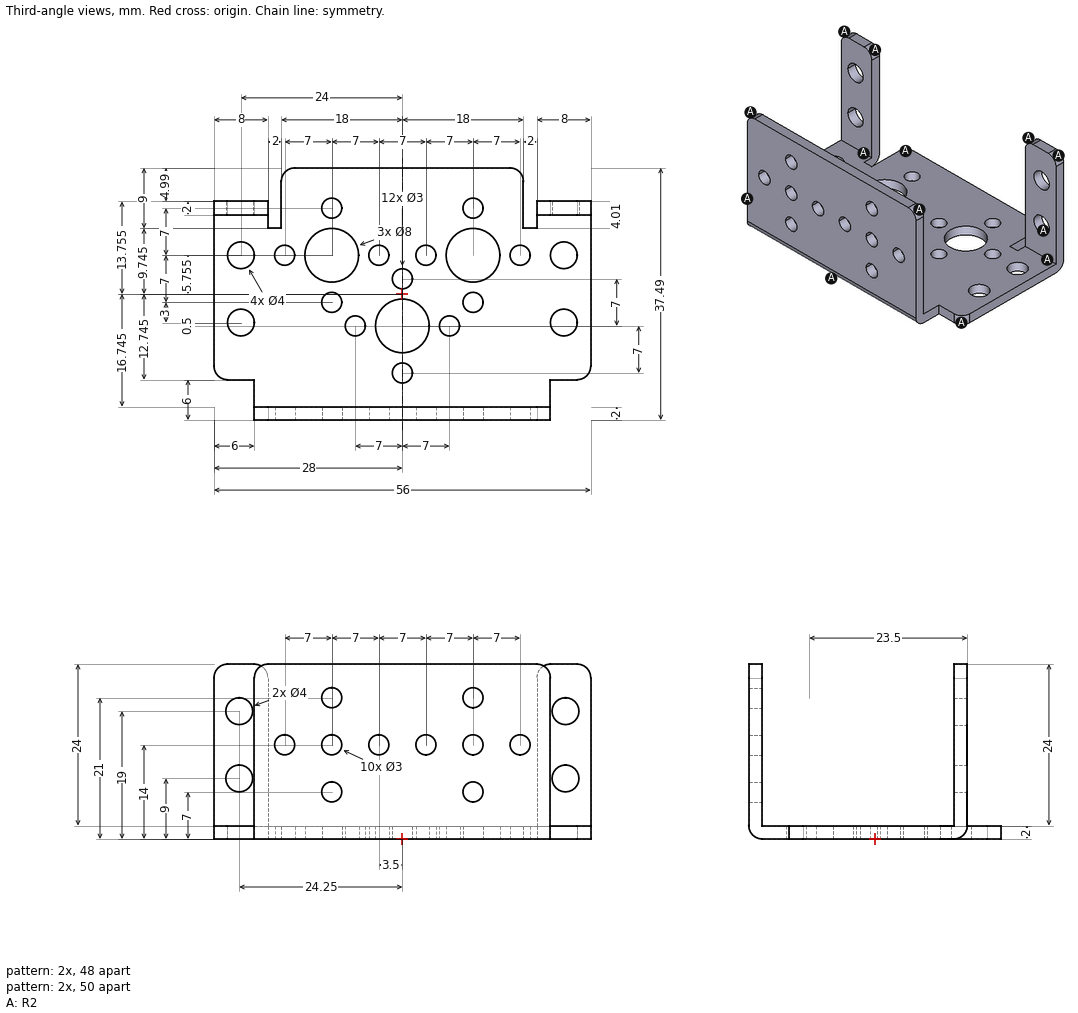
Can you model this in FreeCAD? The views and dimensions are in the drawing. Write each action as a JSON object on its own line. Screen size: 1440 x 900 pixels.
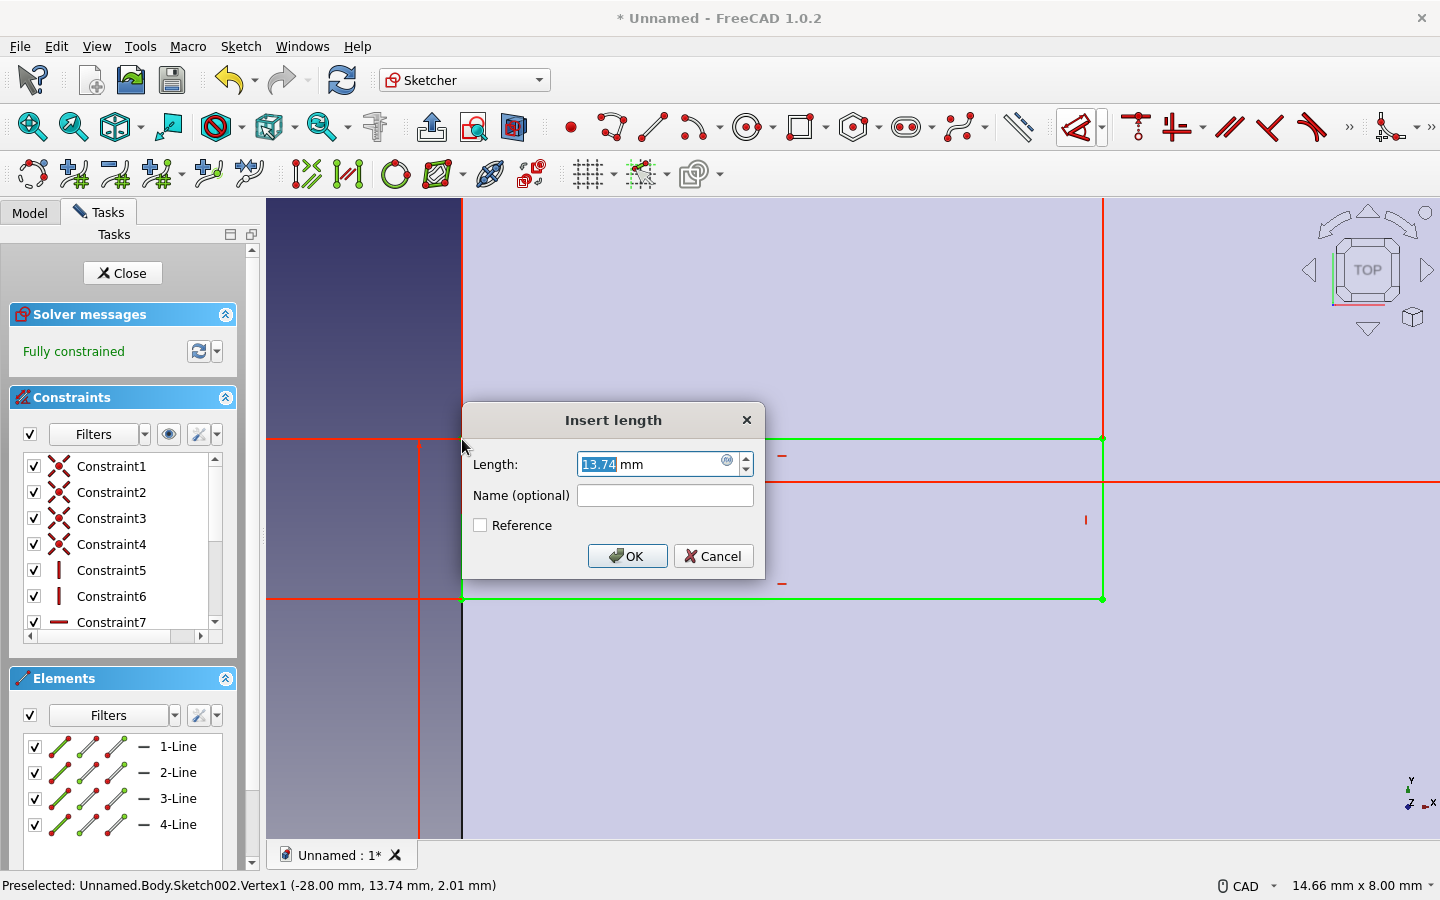
{"action": "type", "text": "13.755"}
{"action": "key", "text": "Return"}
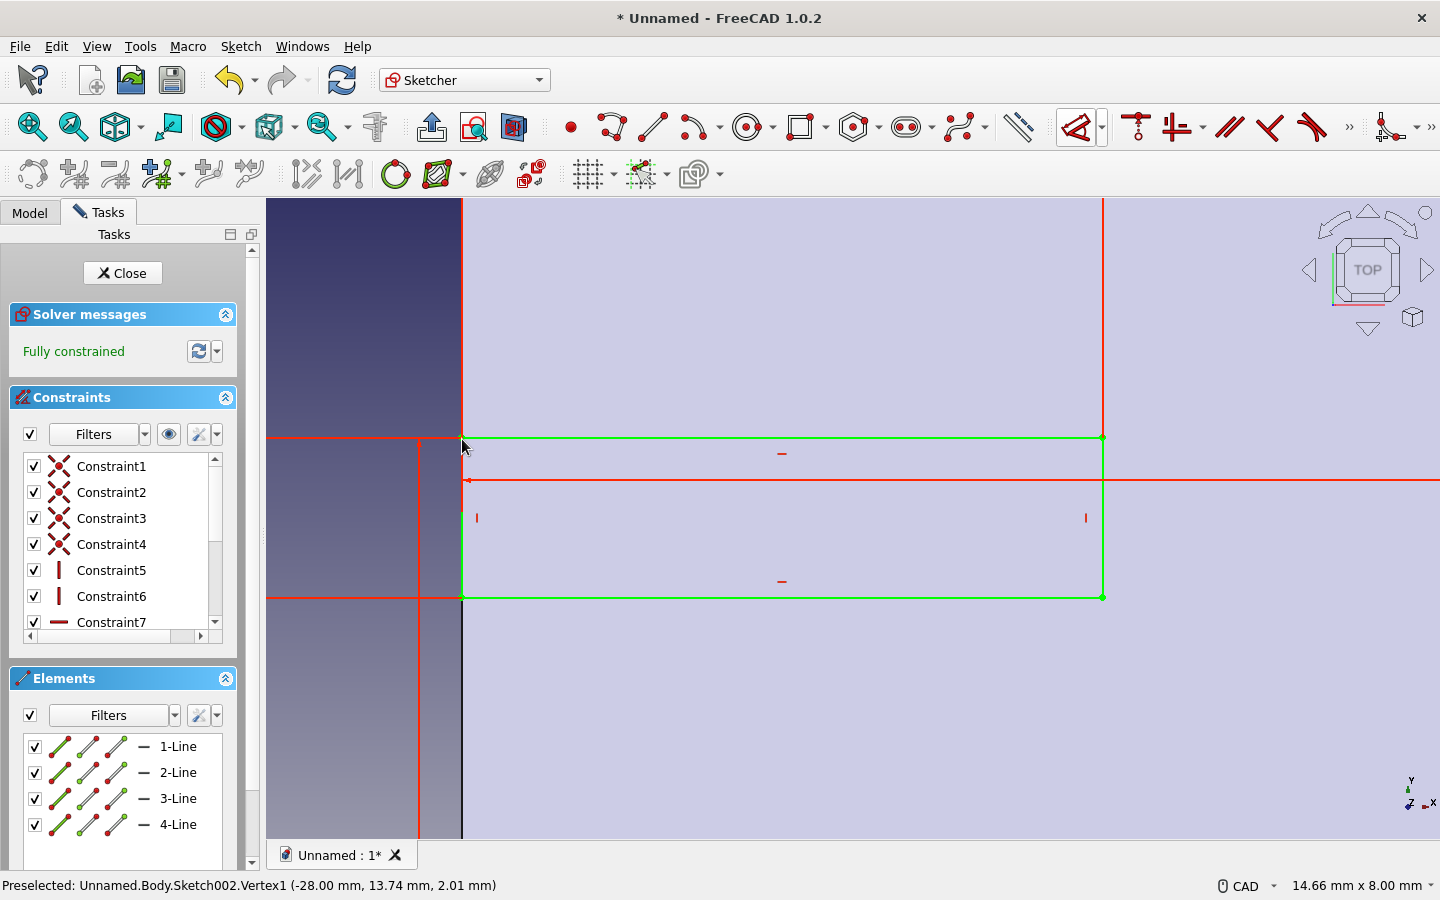
{"action": "left_click", "coordinate": [123, 273]}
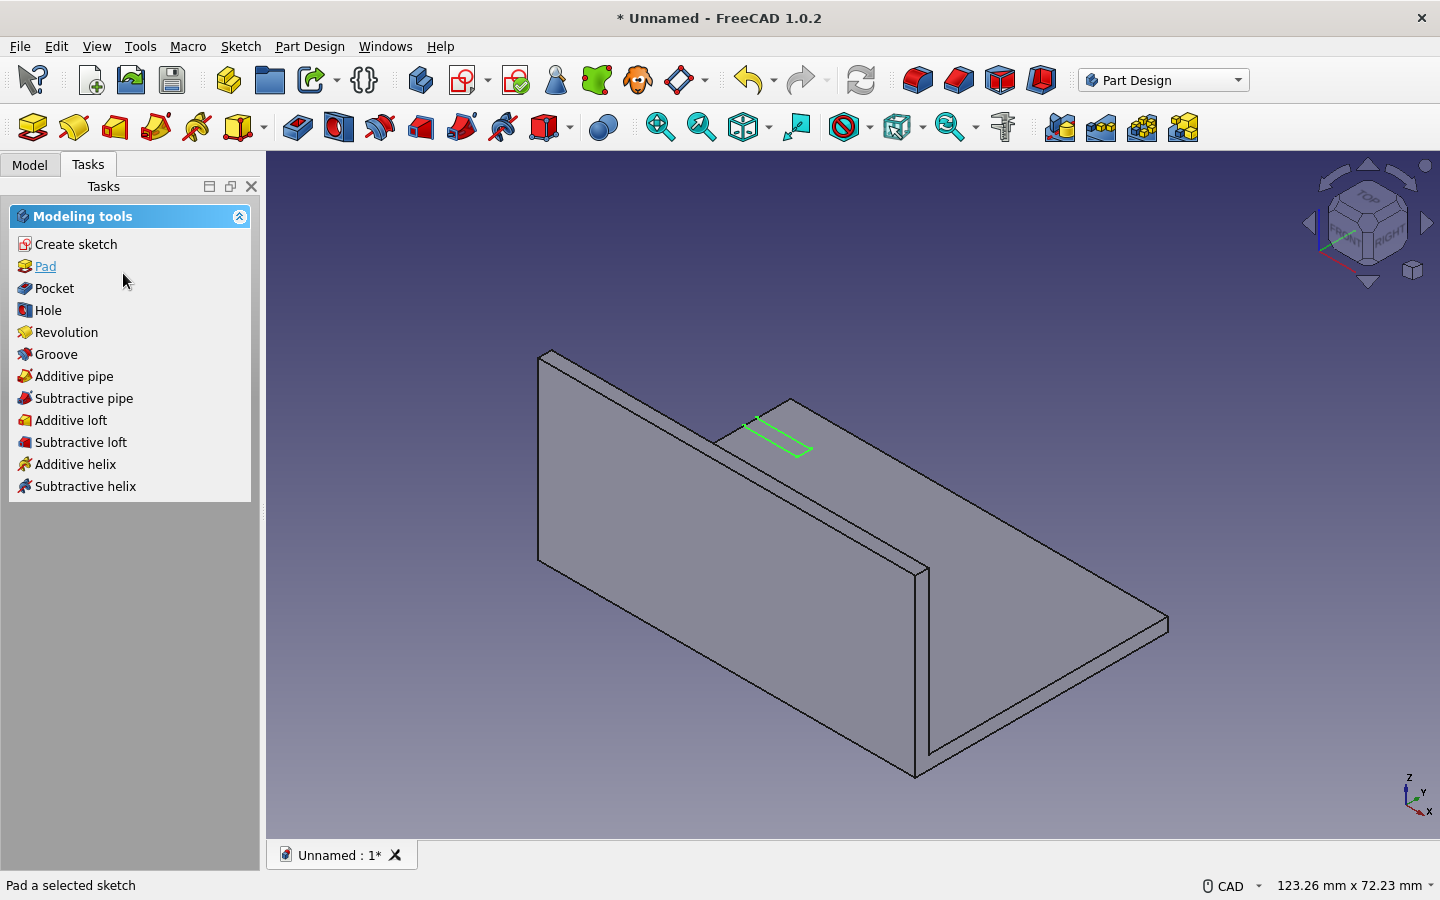
{"action": "left_click", "coordinate": [33, 128]}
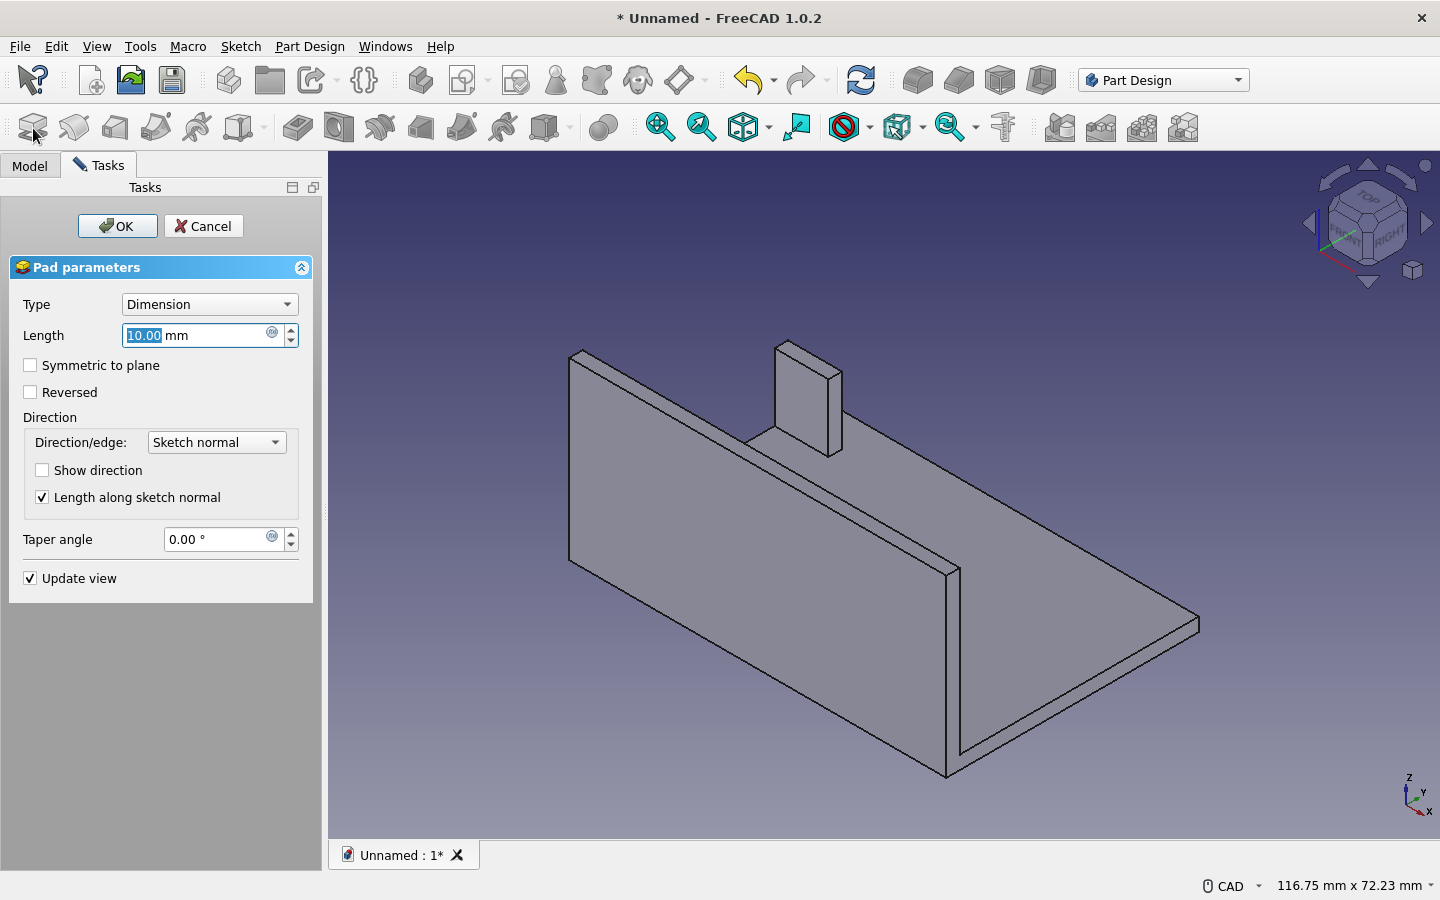
{"action": "type", "text": "24"}
{"action": "key", "text": "Tab"}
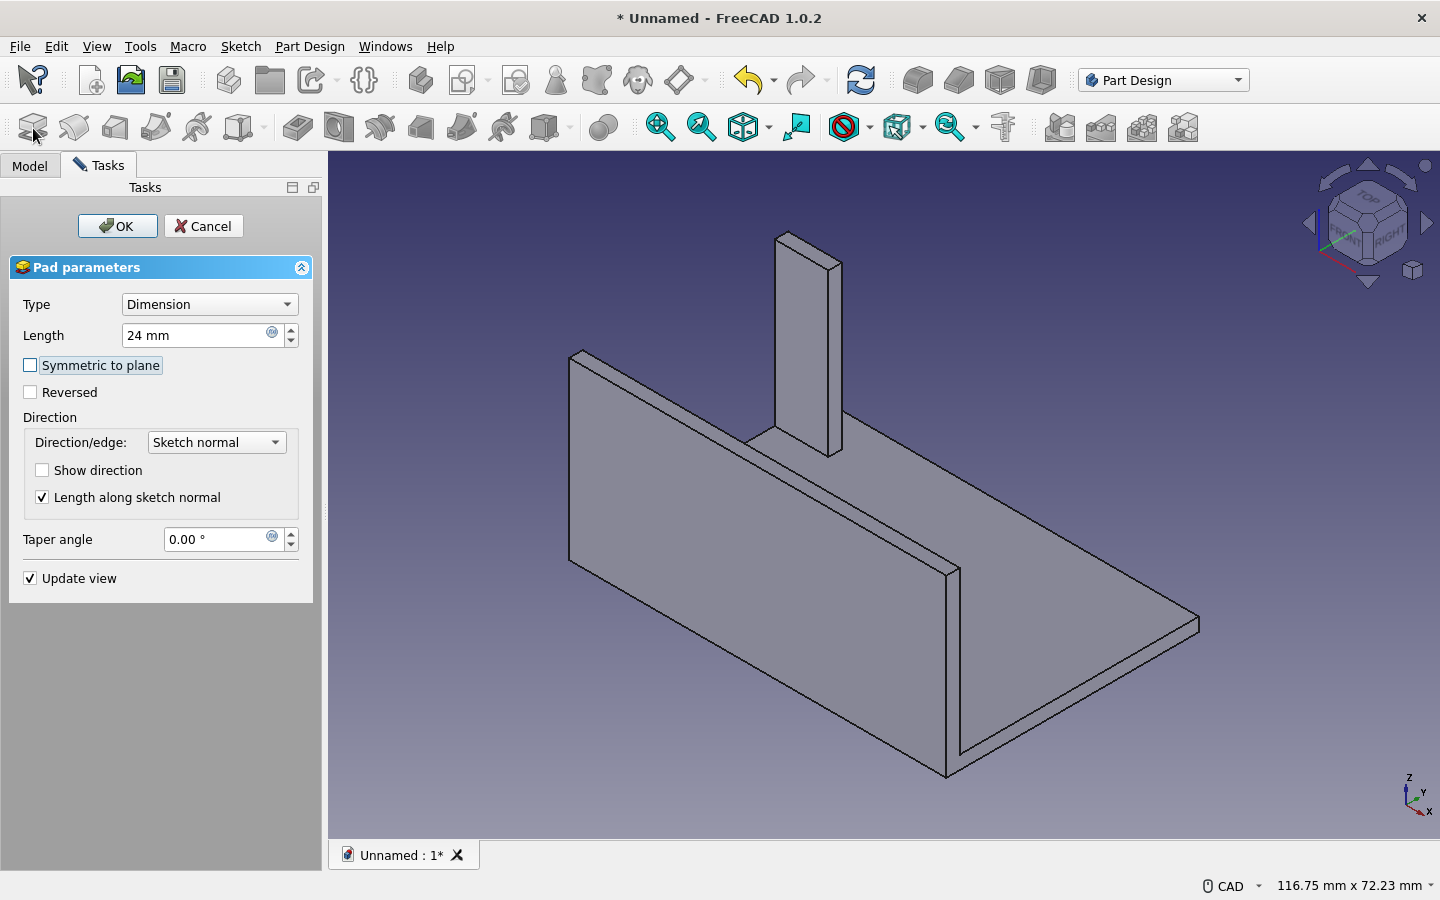
{"action": "left_click", "coordinate": [118, 226]}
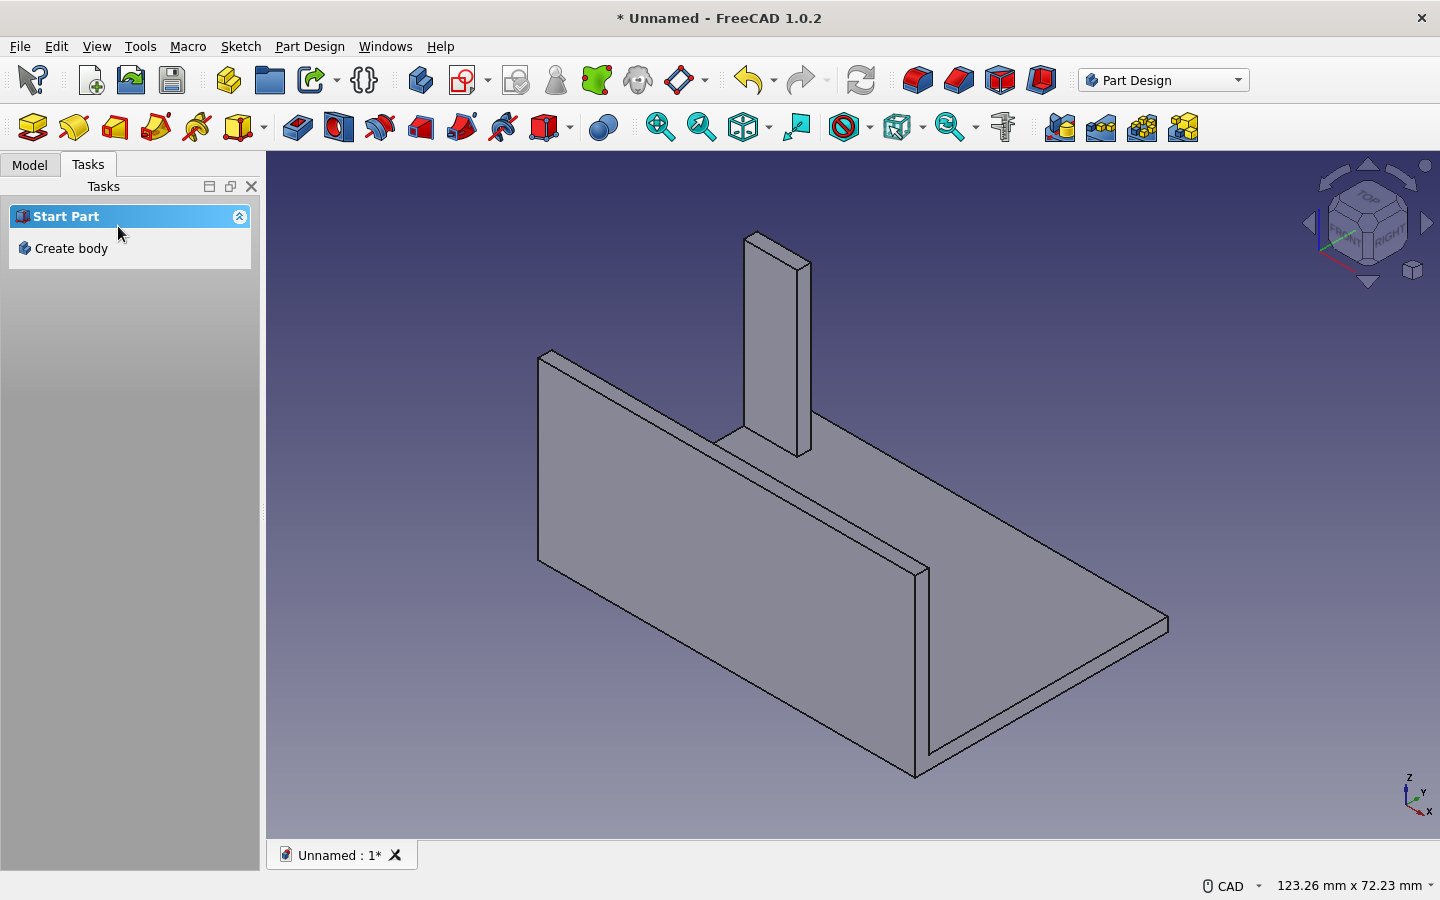
{"action": "left_click", "coordinate": [30, 164]}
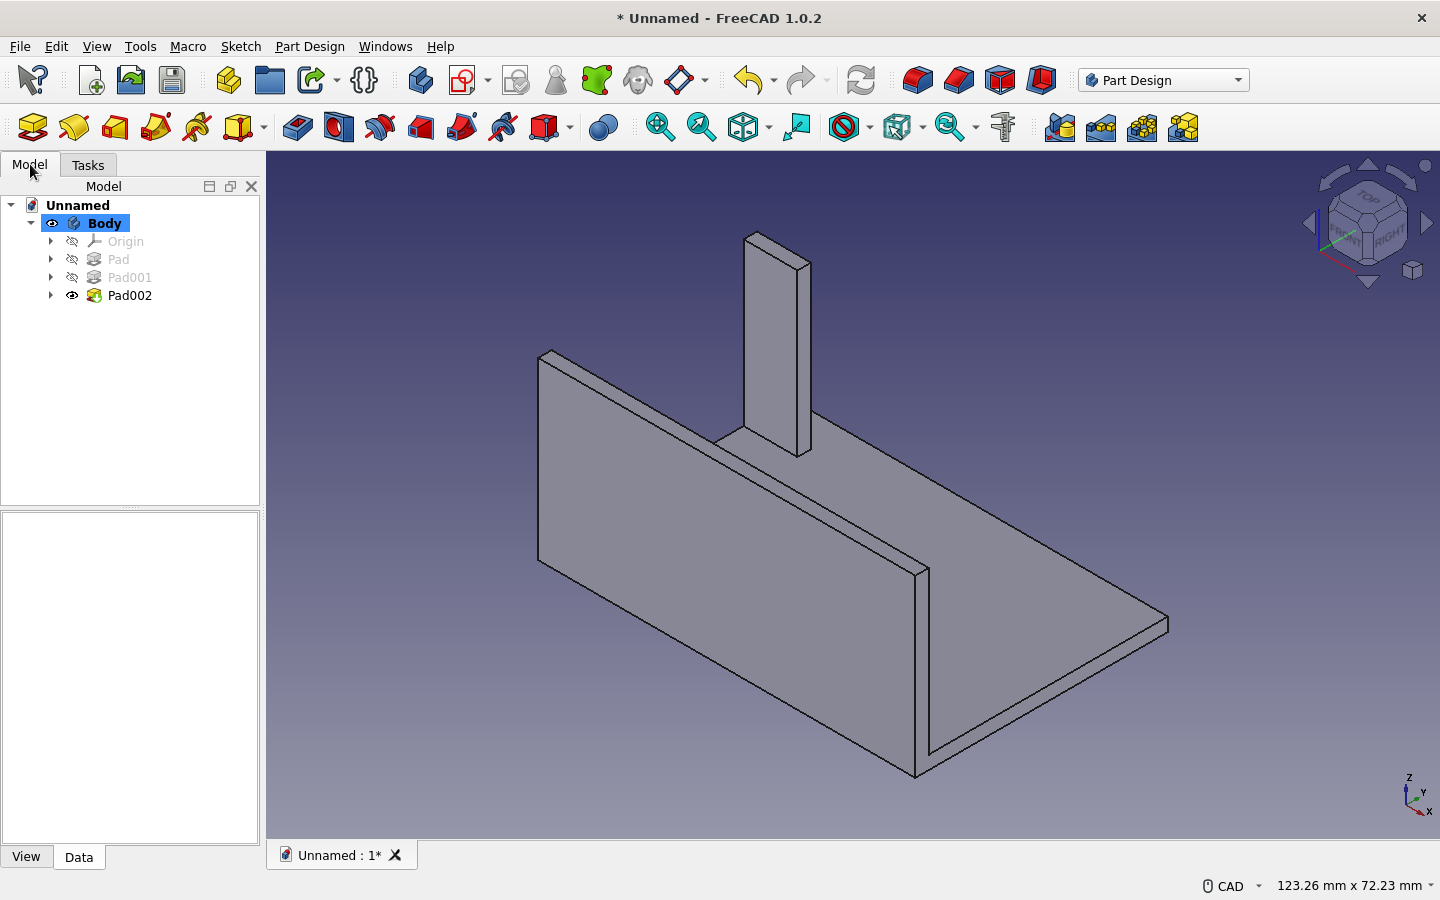
{"action": "left_click", "coordinate": [117, 295]}